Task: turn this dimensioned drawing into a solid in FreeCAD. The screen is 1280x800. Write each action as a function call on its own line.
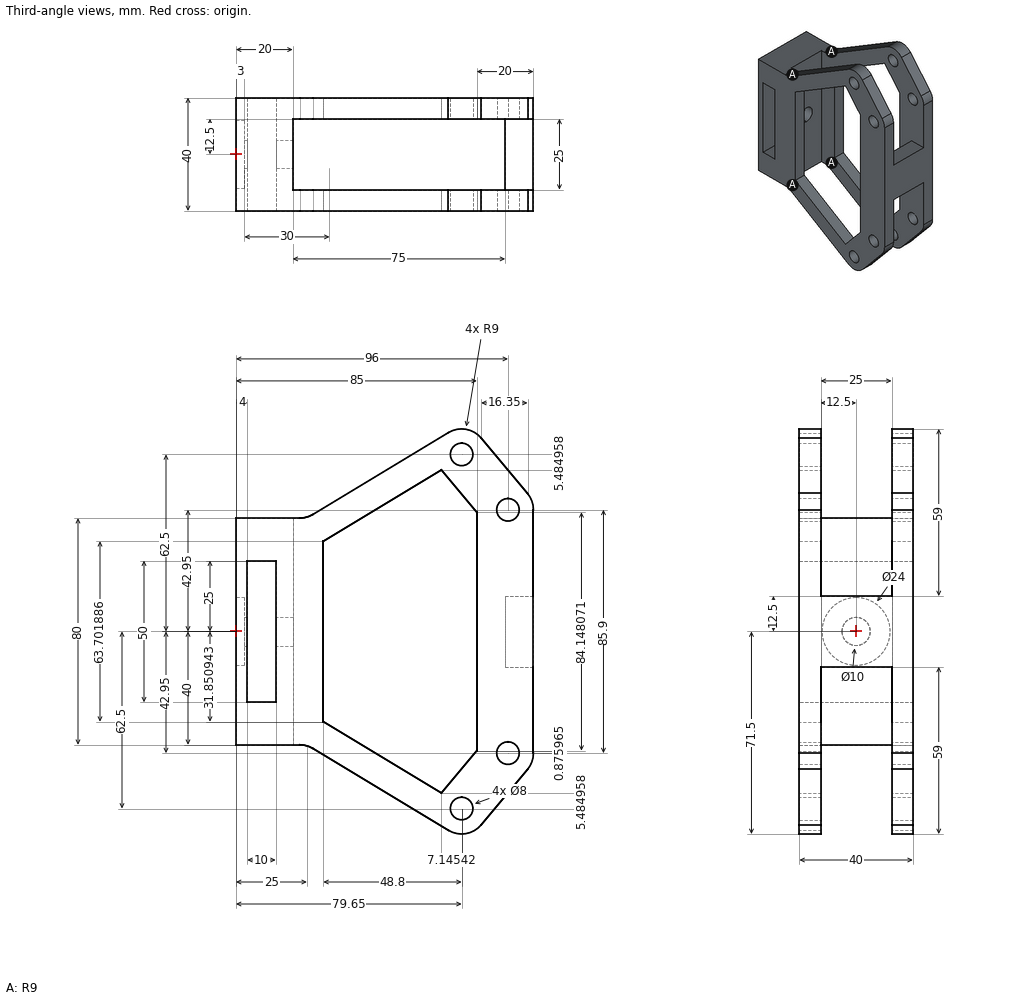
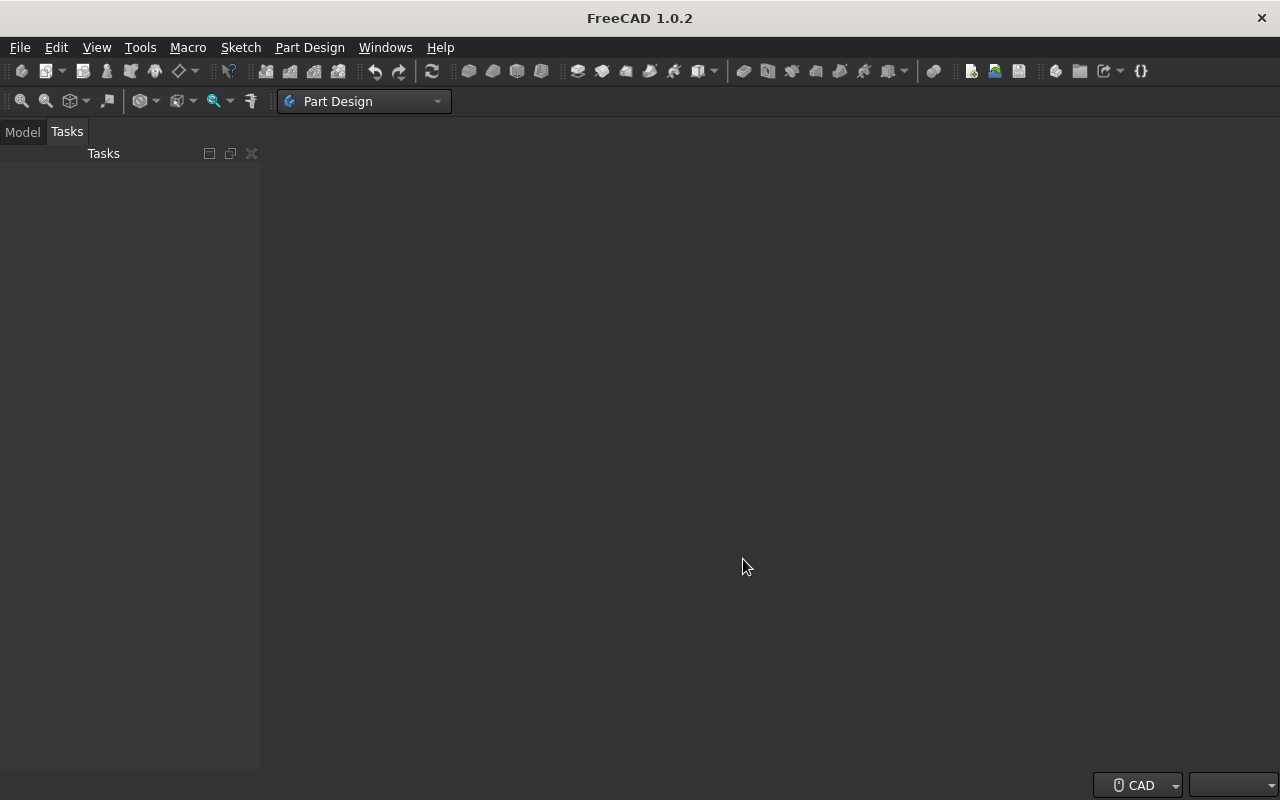
key(ctrl+n)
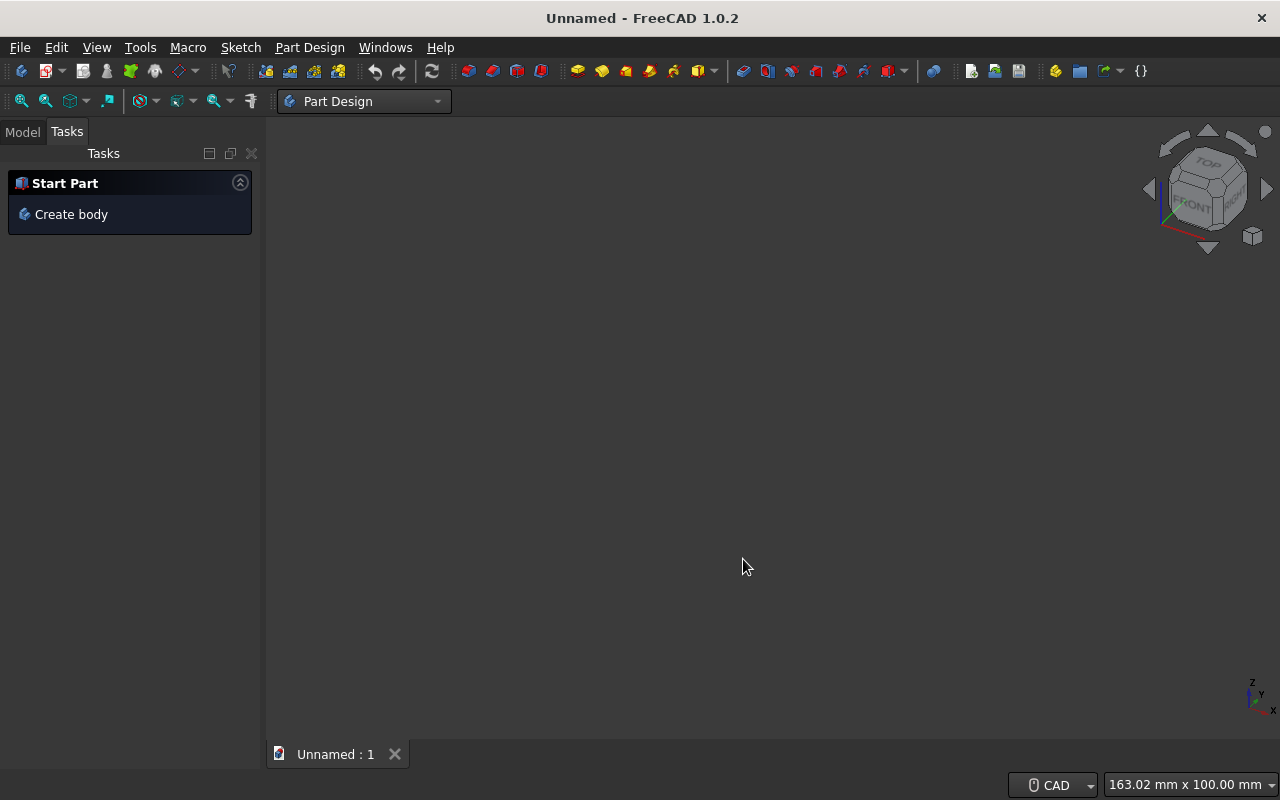
click(46, 72)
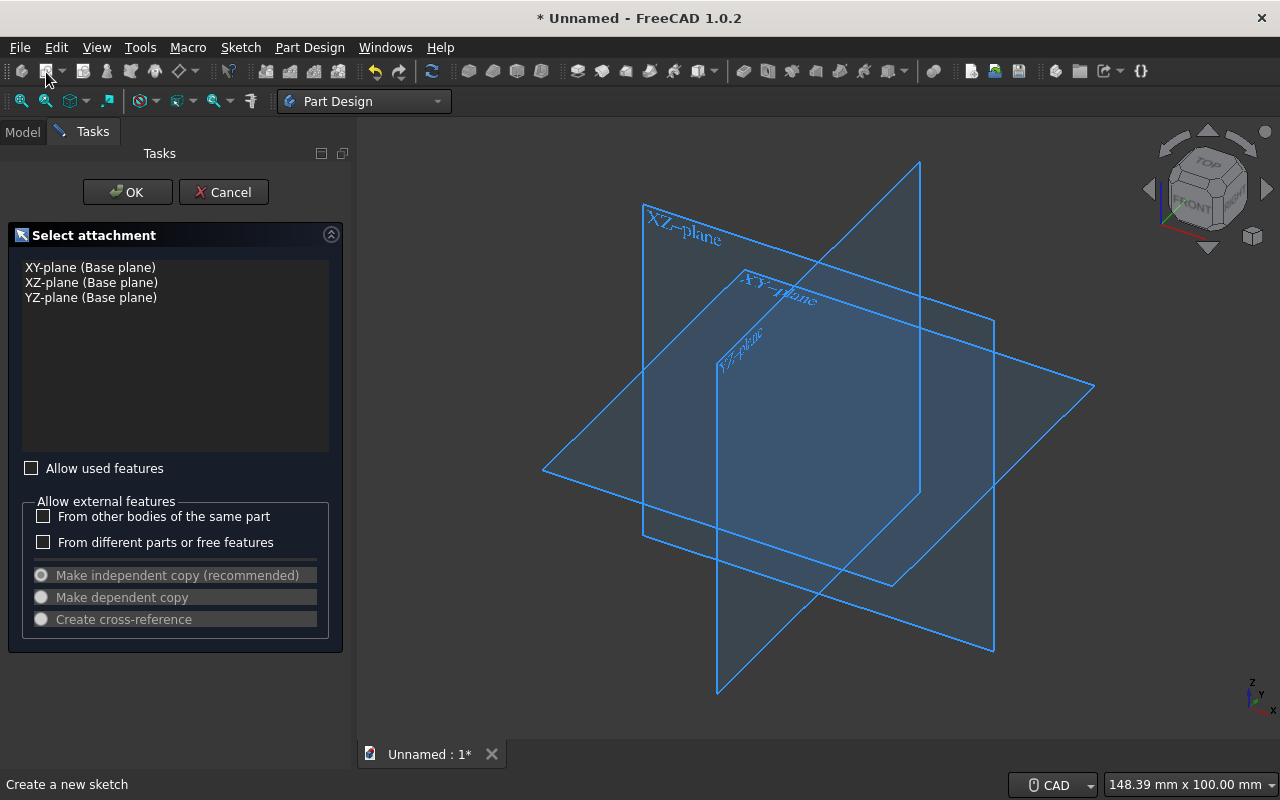
click(82, 282)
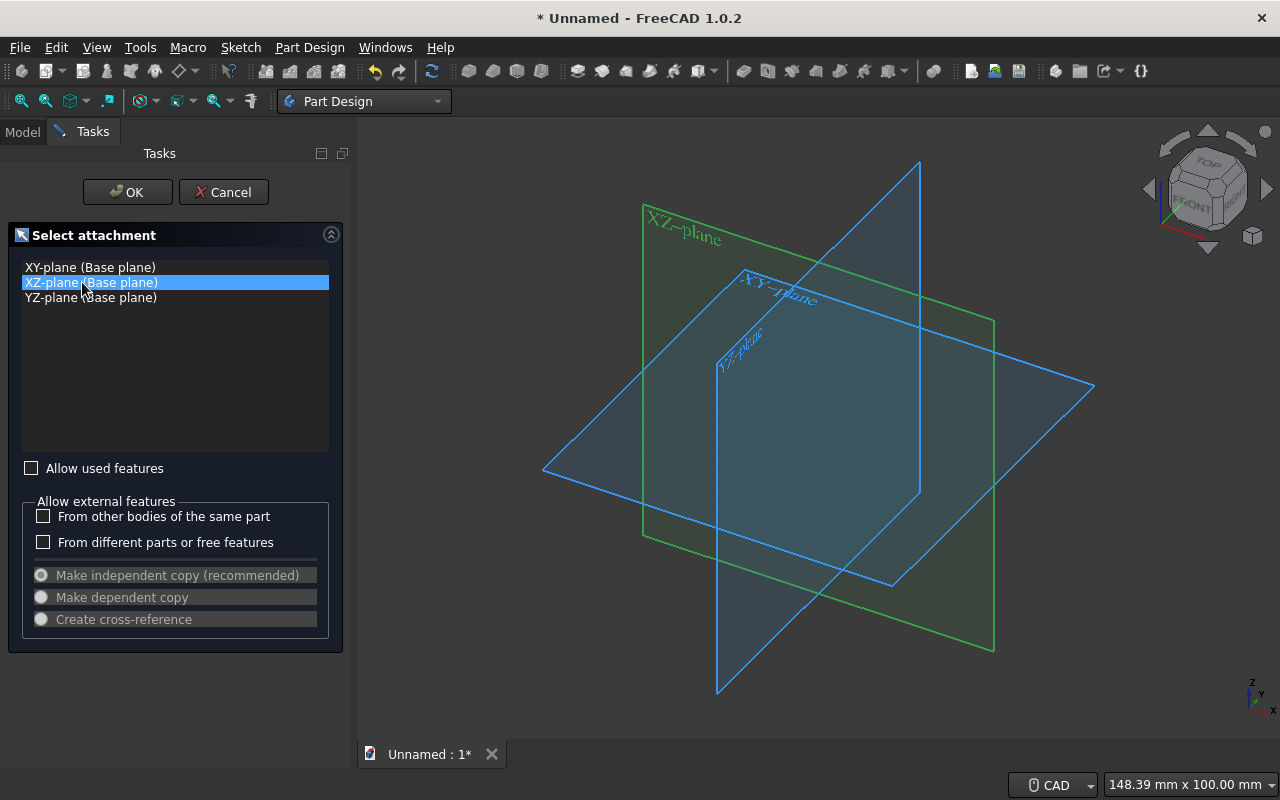
click(128, 192)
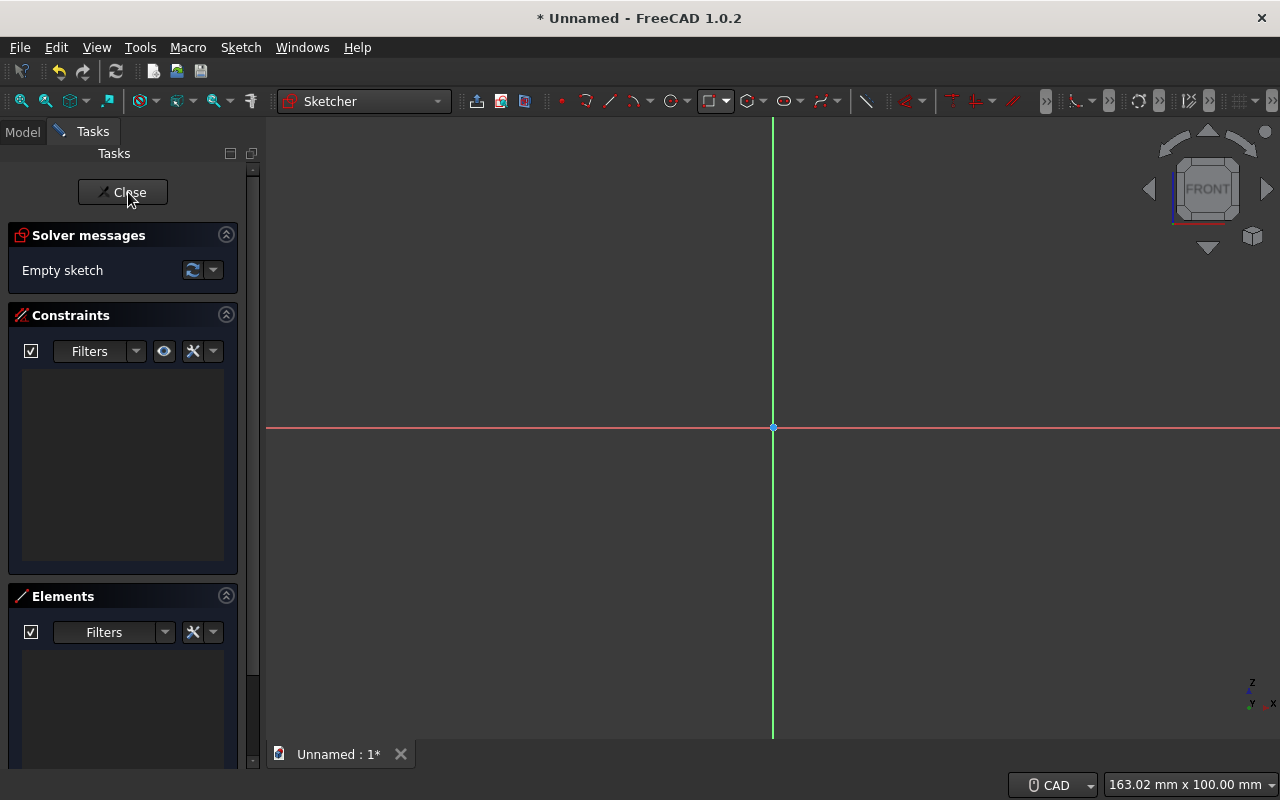
scroll(382, 428, down, 4)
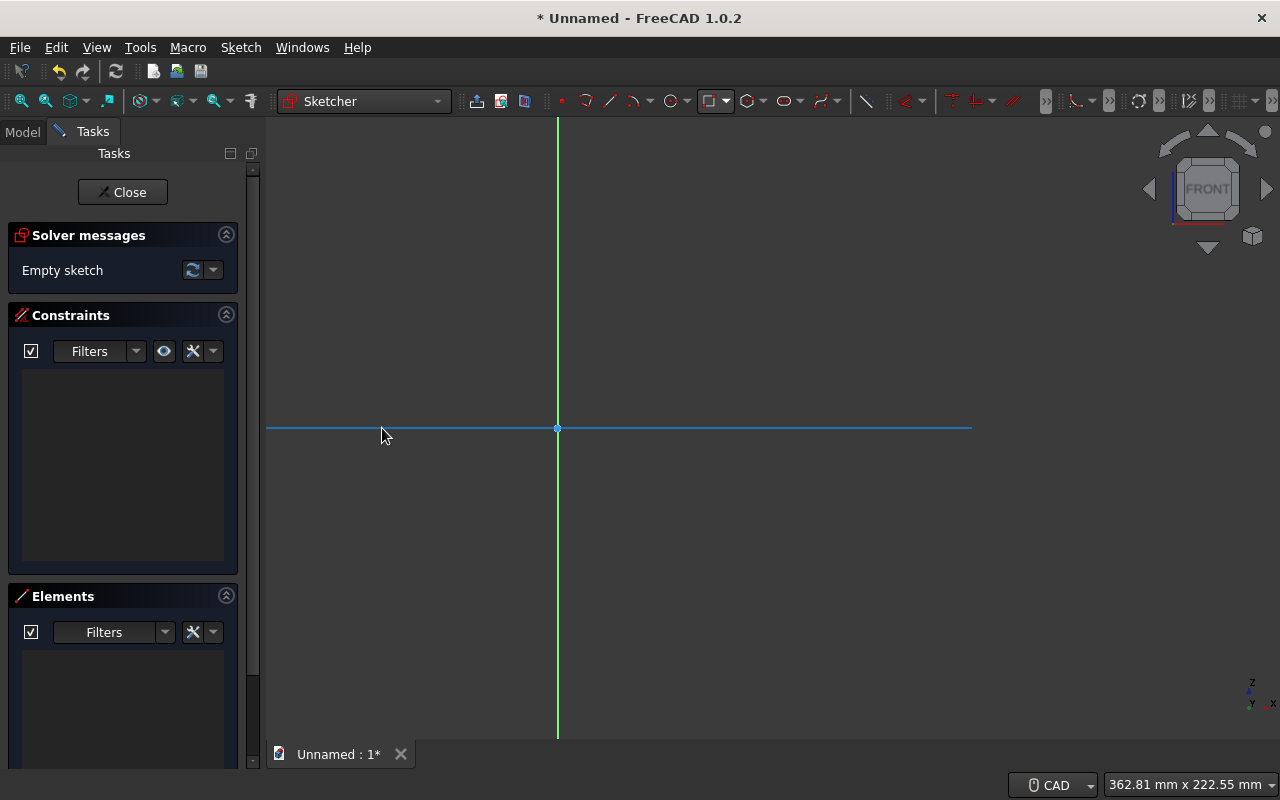
click(586, 102)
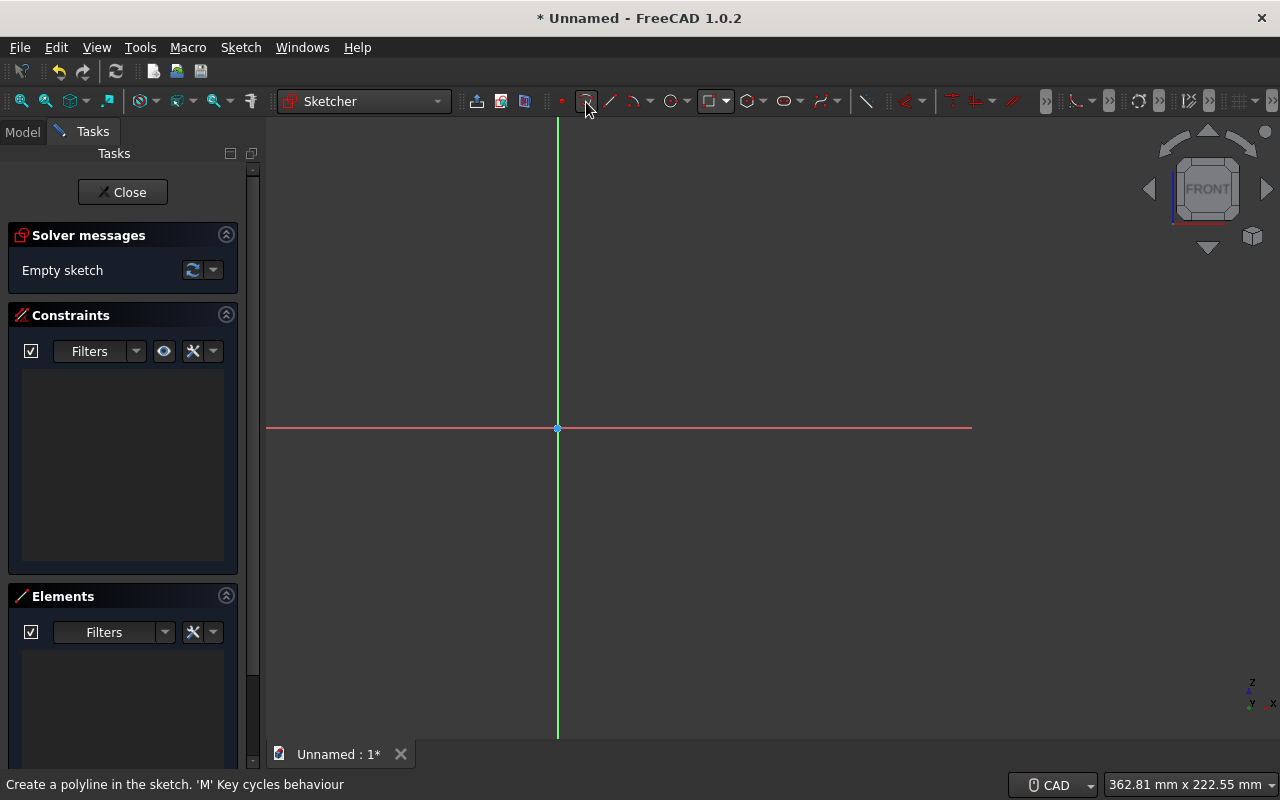
click(767, 624)
click(628, 540)
click(558, 540)
click(567, 316)
click(628, 316)
click(767, 232)
right_click(767, 232)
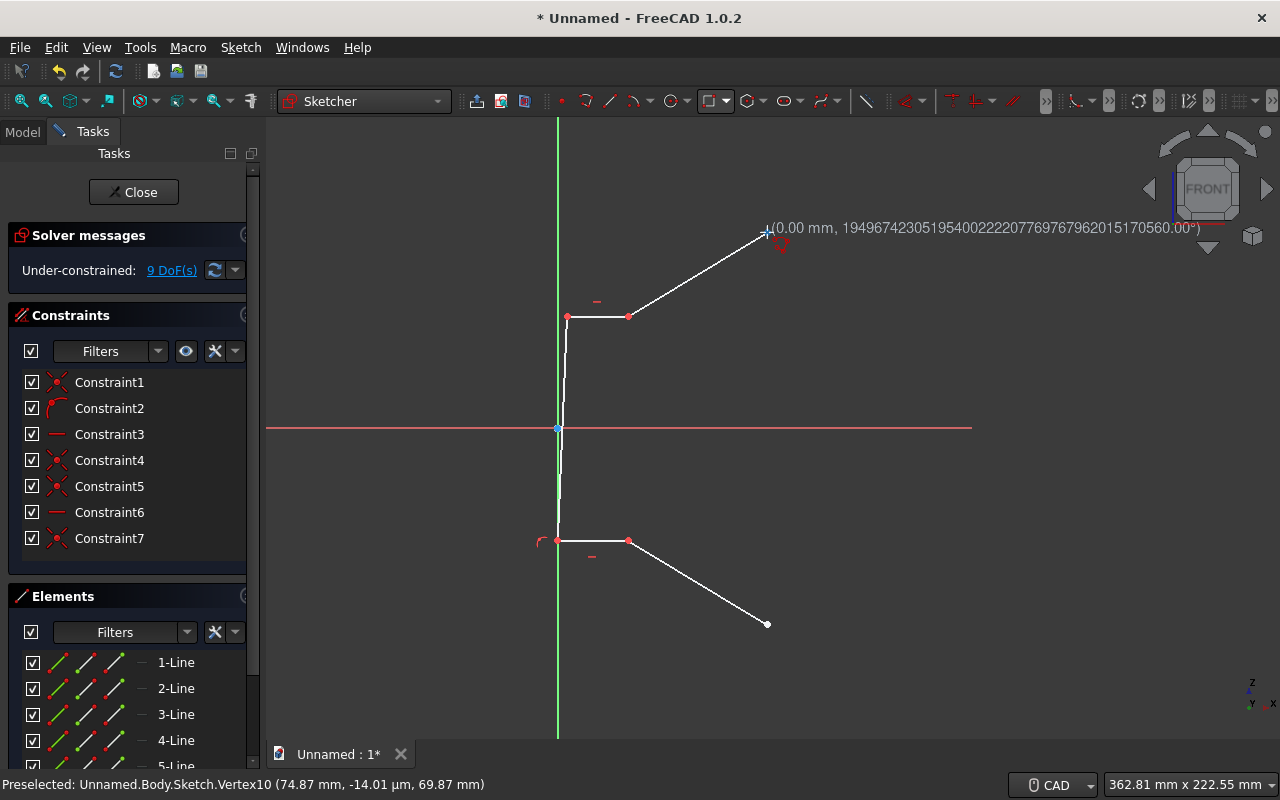
key(g)
key(l)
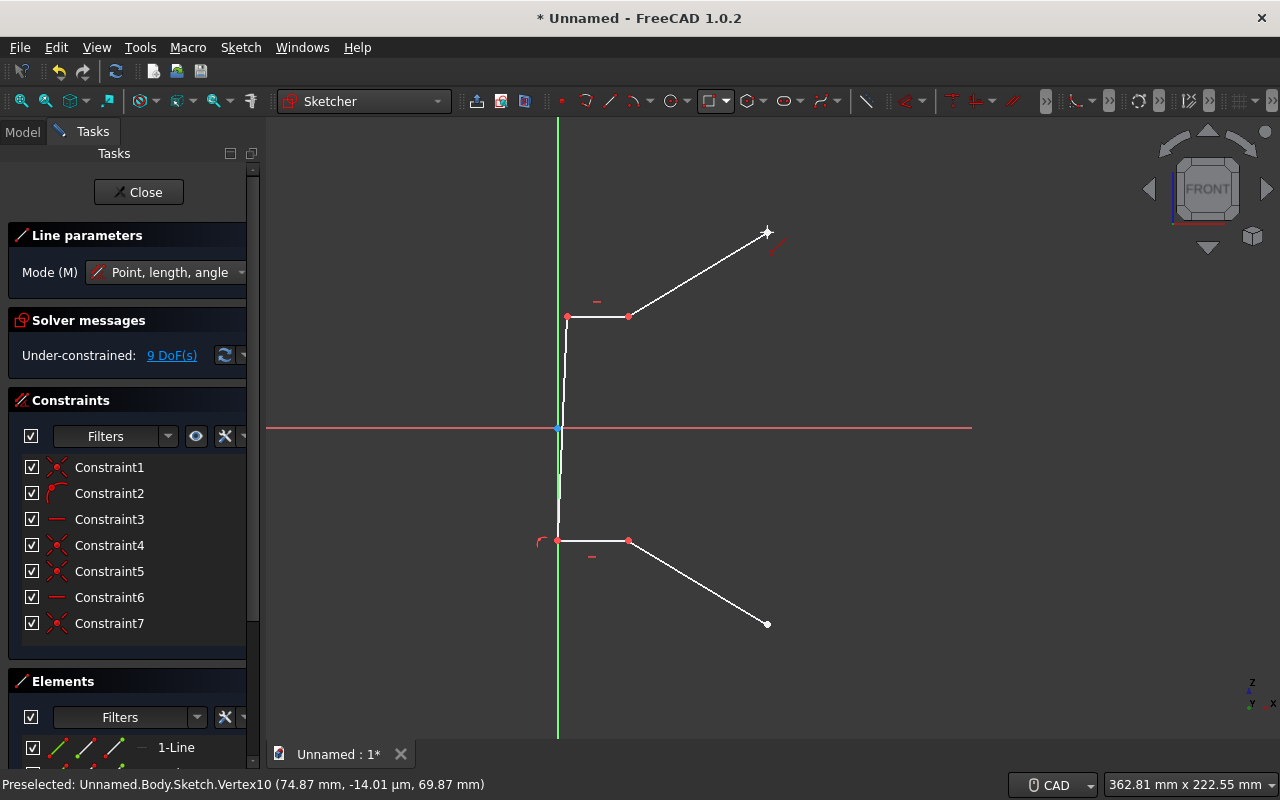
click(800, 237)
click(845, 292)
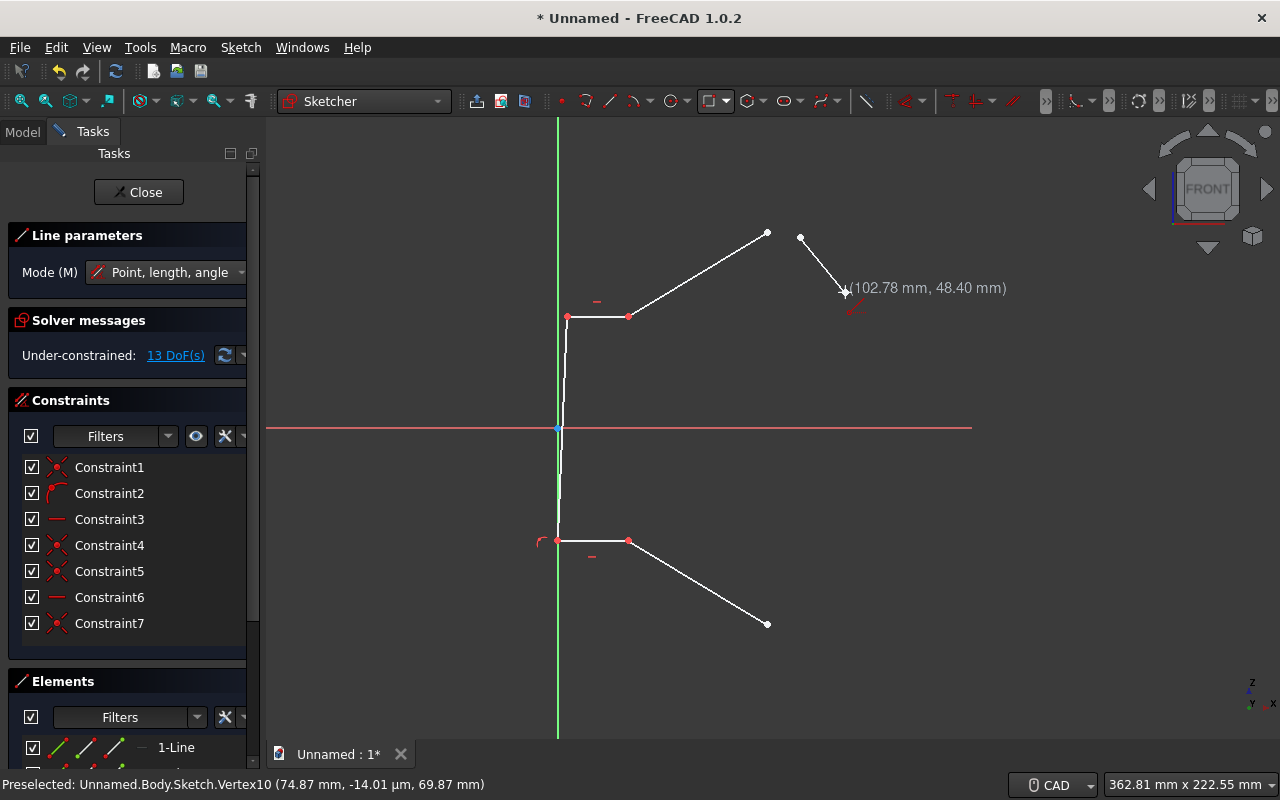
click(851, 308)
click(851, 548)